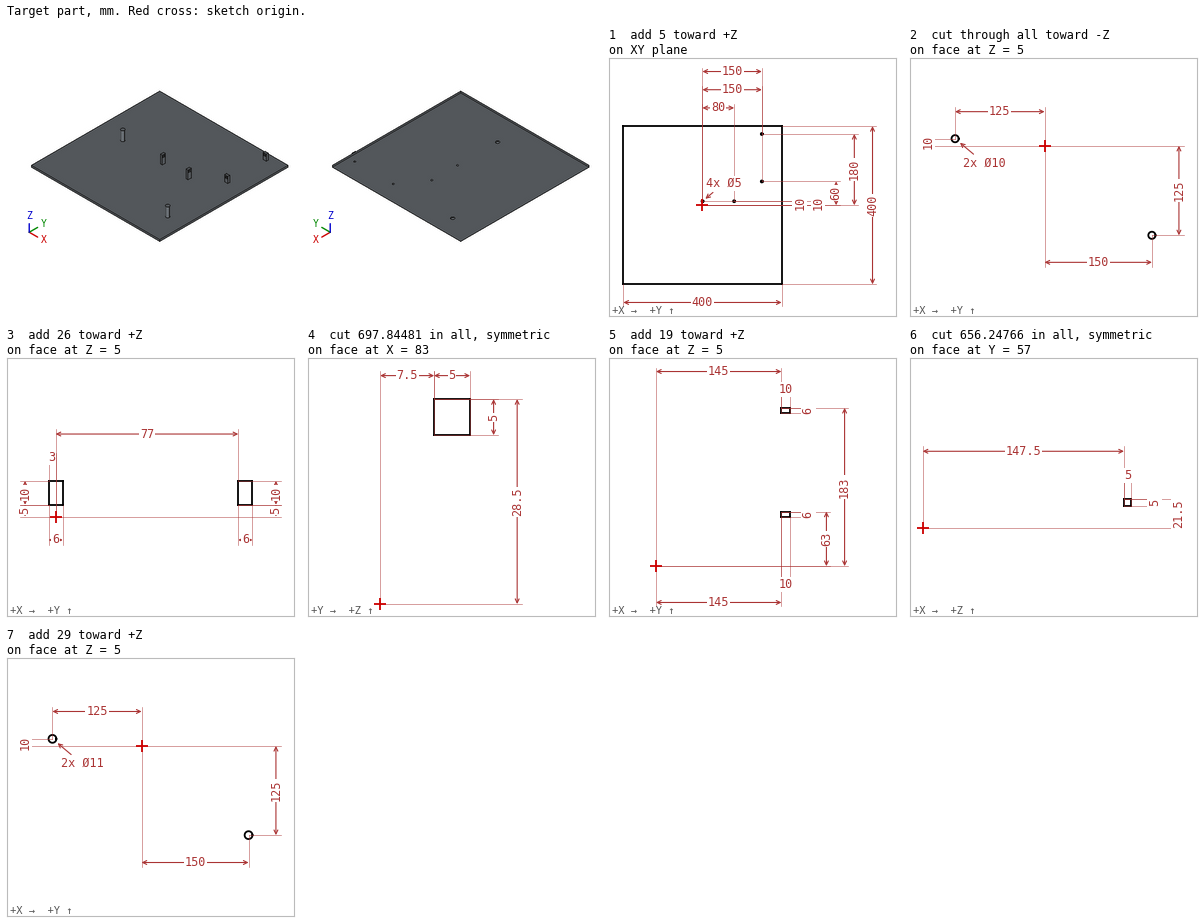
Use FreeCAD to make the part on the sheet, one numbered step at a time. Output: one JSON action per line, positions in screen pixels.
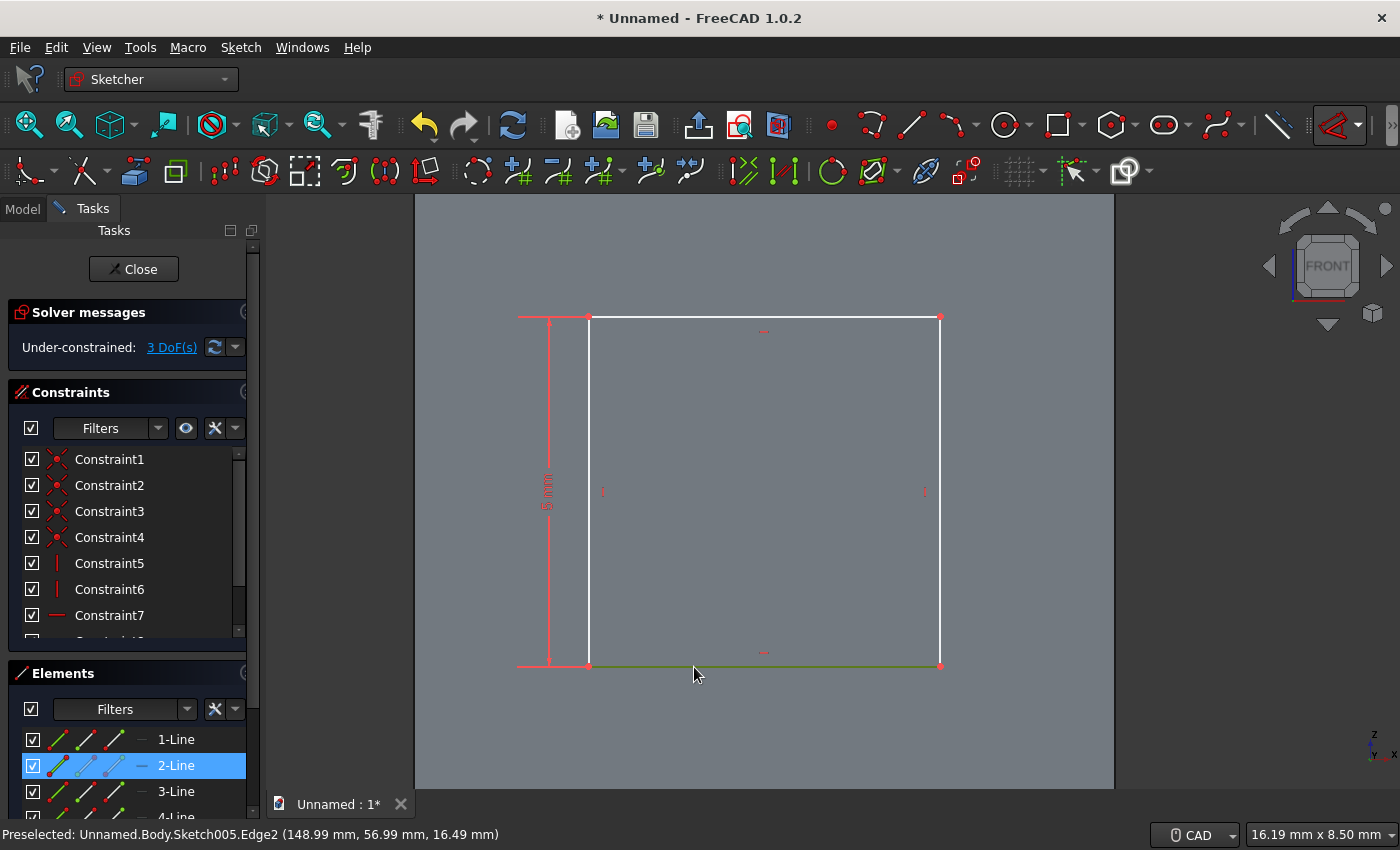
{"action": "left_click", "coordinate": [1360, 126]}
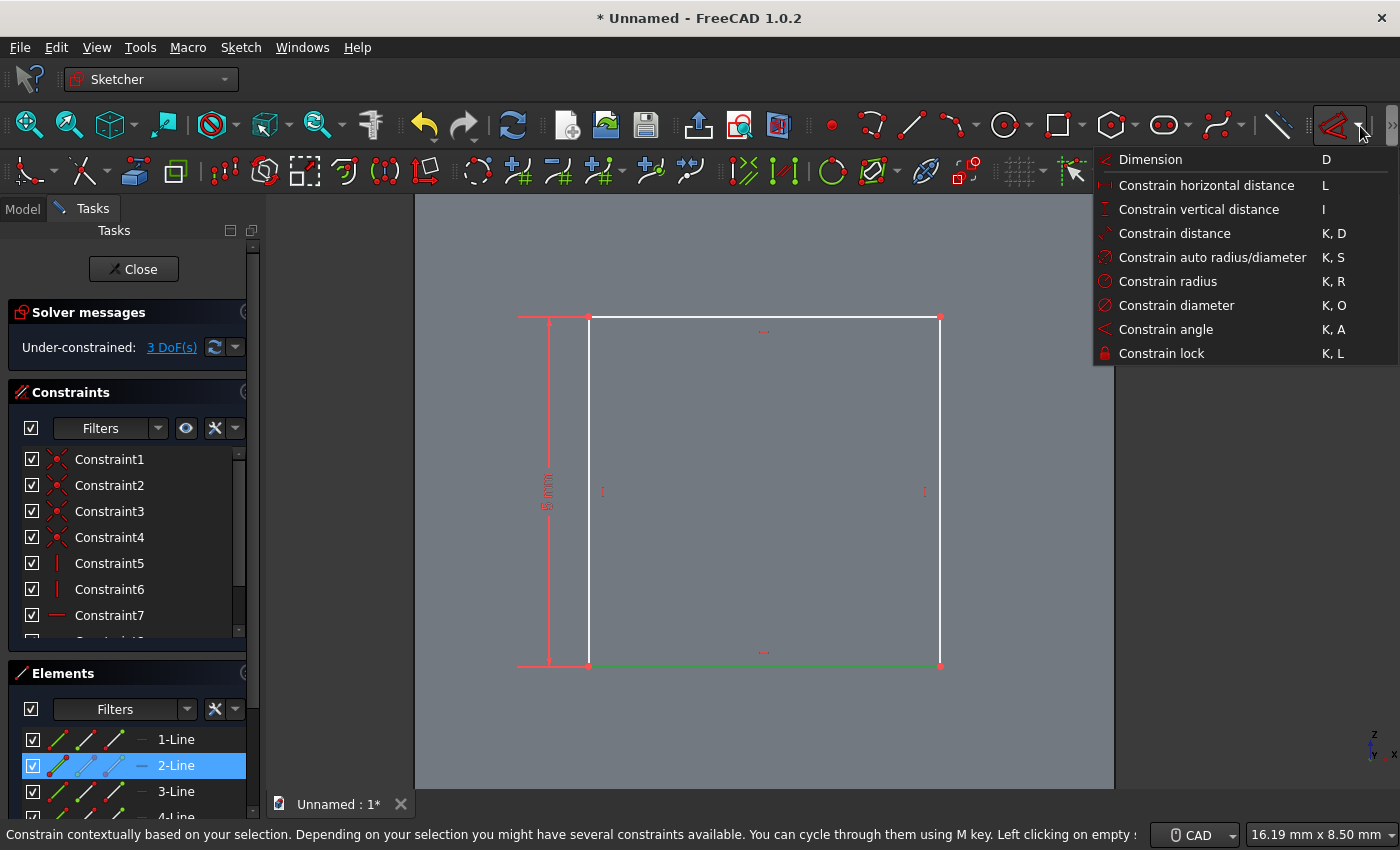
{"action": "left_click", "coordinate": [1246, 185]}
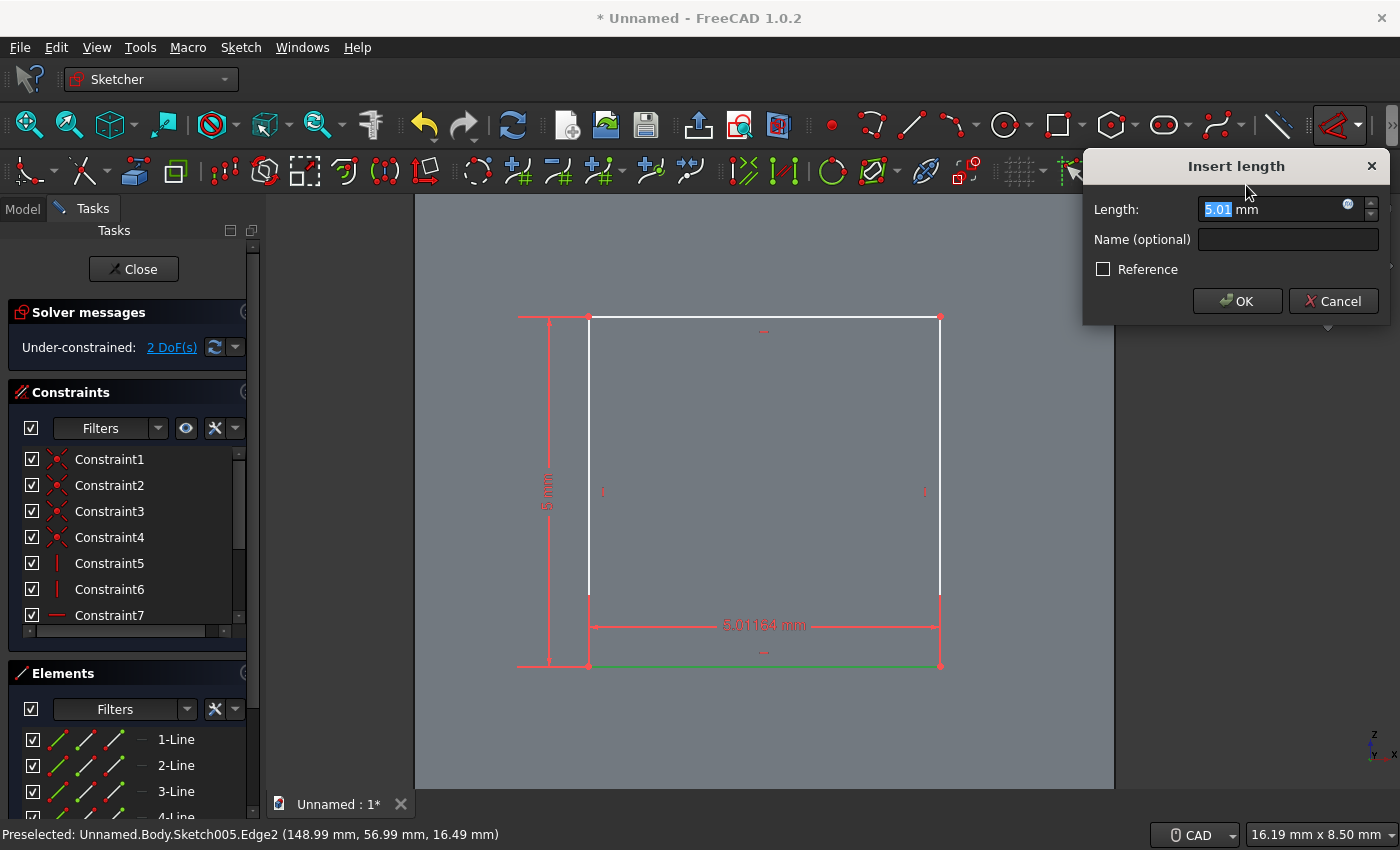
{"action": "type", "text": "5"}
{"action": "key", "text": "Return"}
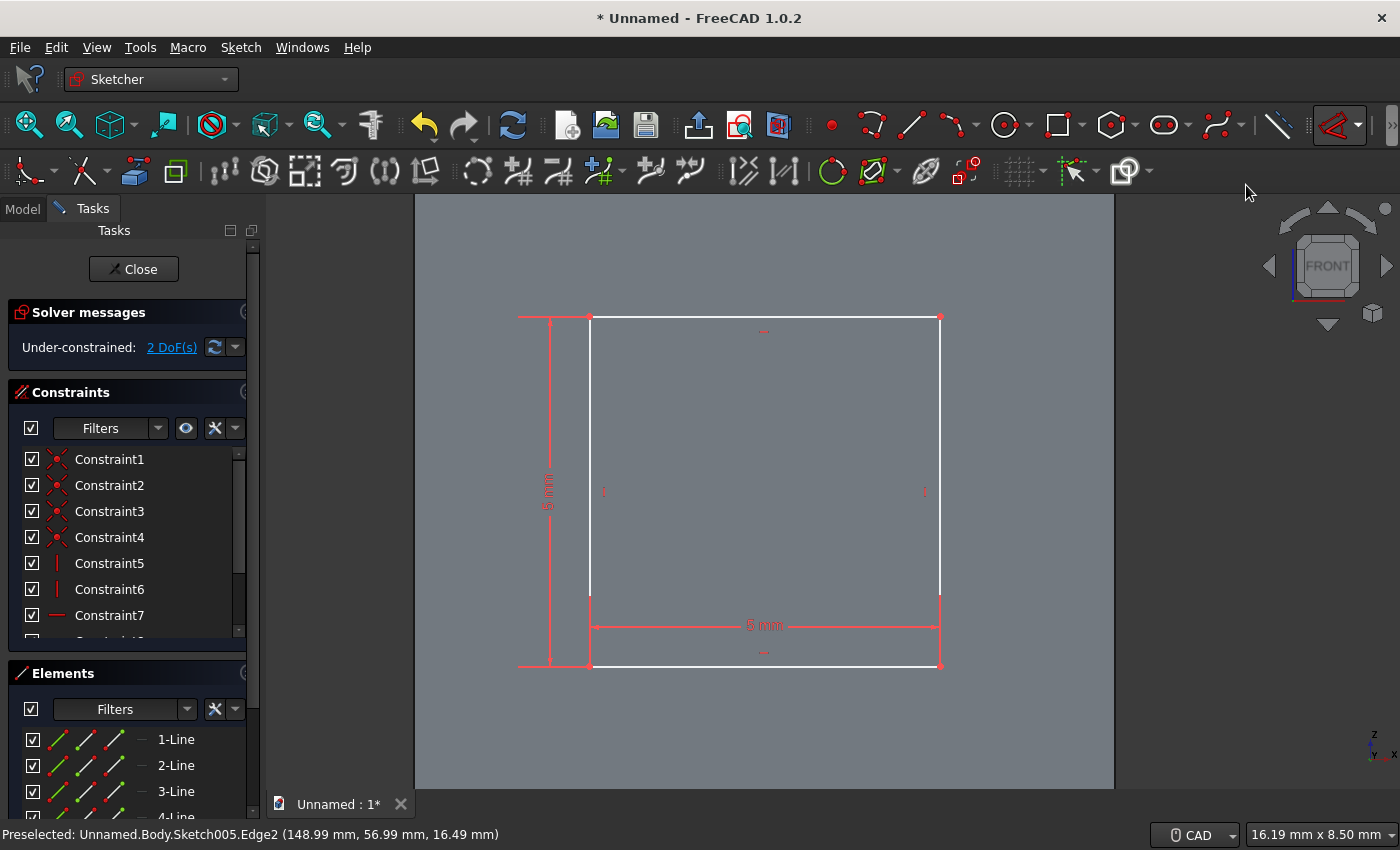
{"action": "left_click", "coordinate": [590, 317]}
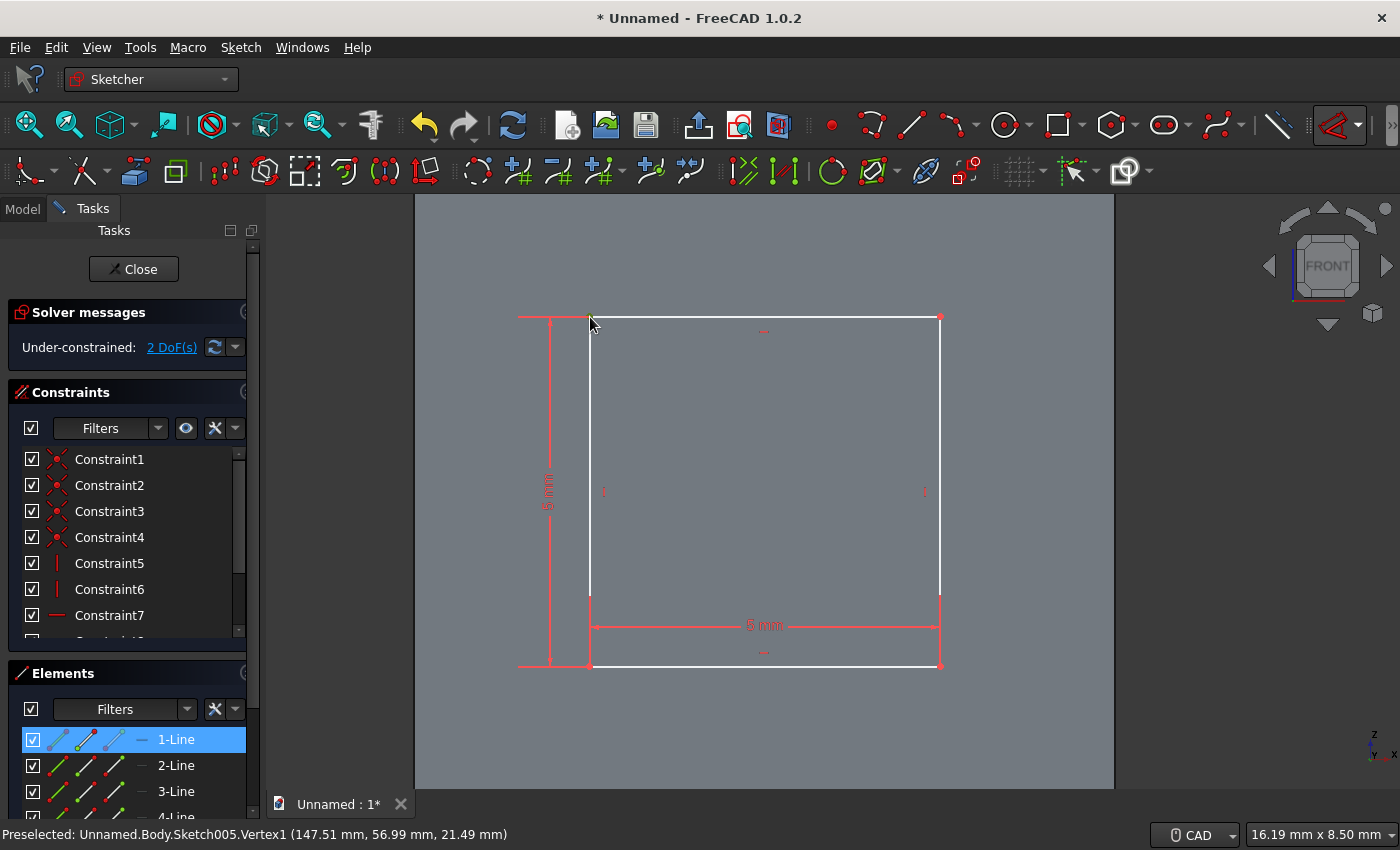
{"action": "key", "text": "i"}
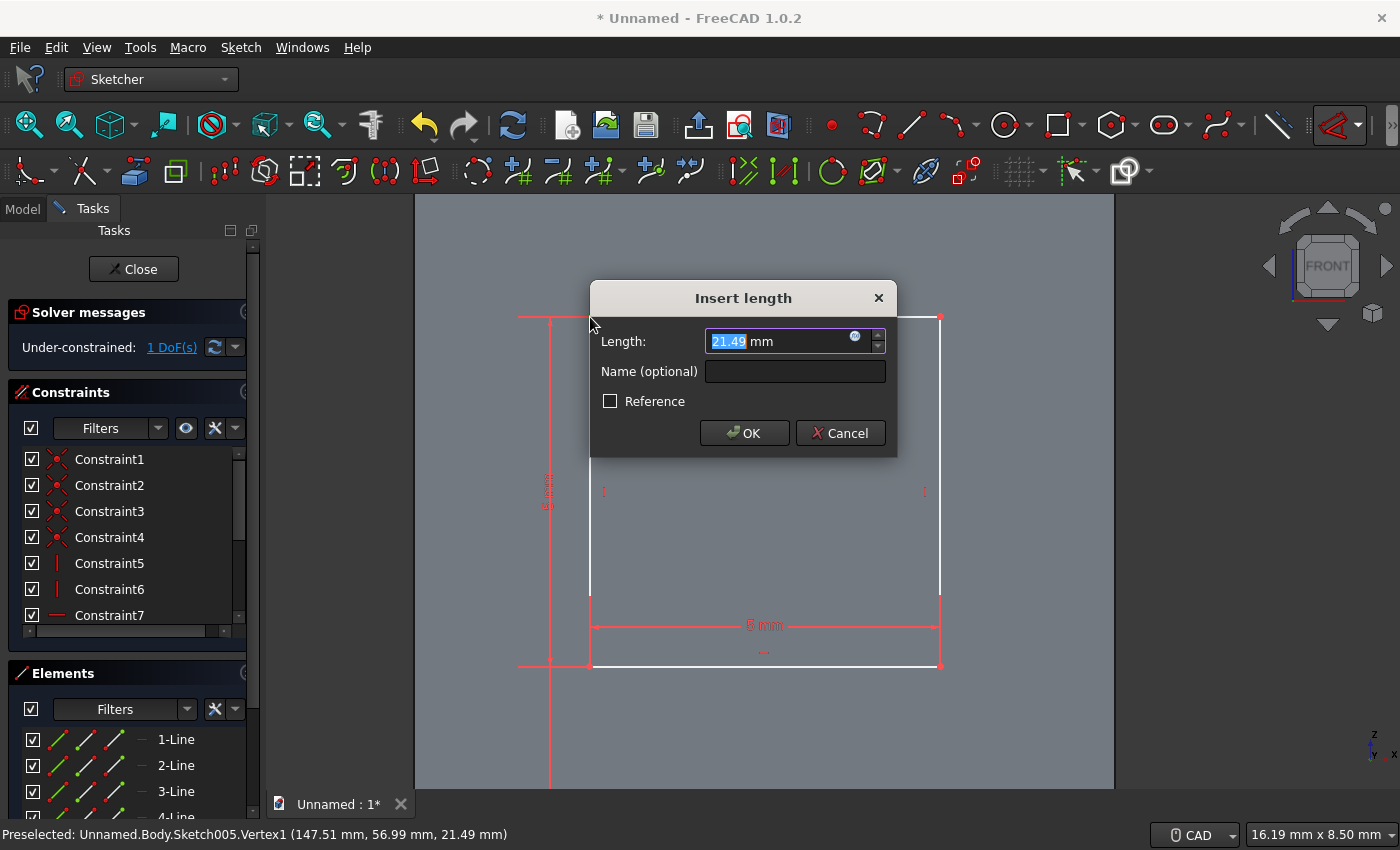
{"action": "type", "text": "21.5"}
{"action": "key", "text": "Return"}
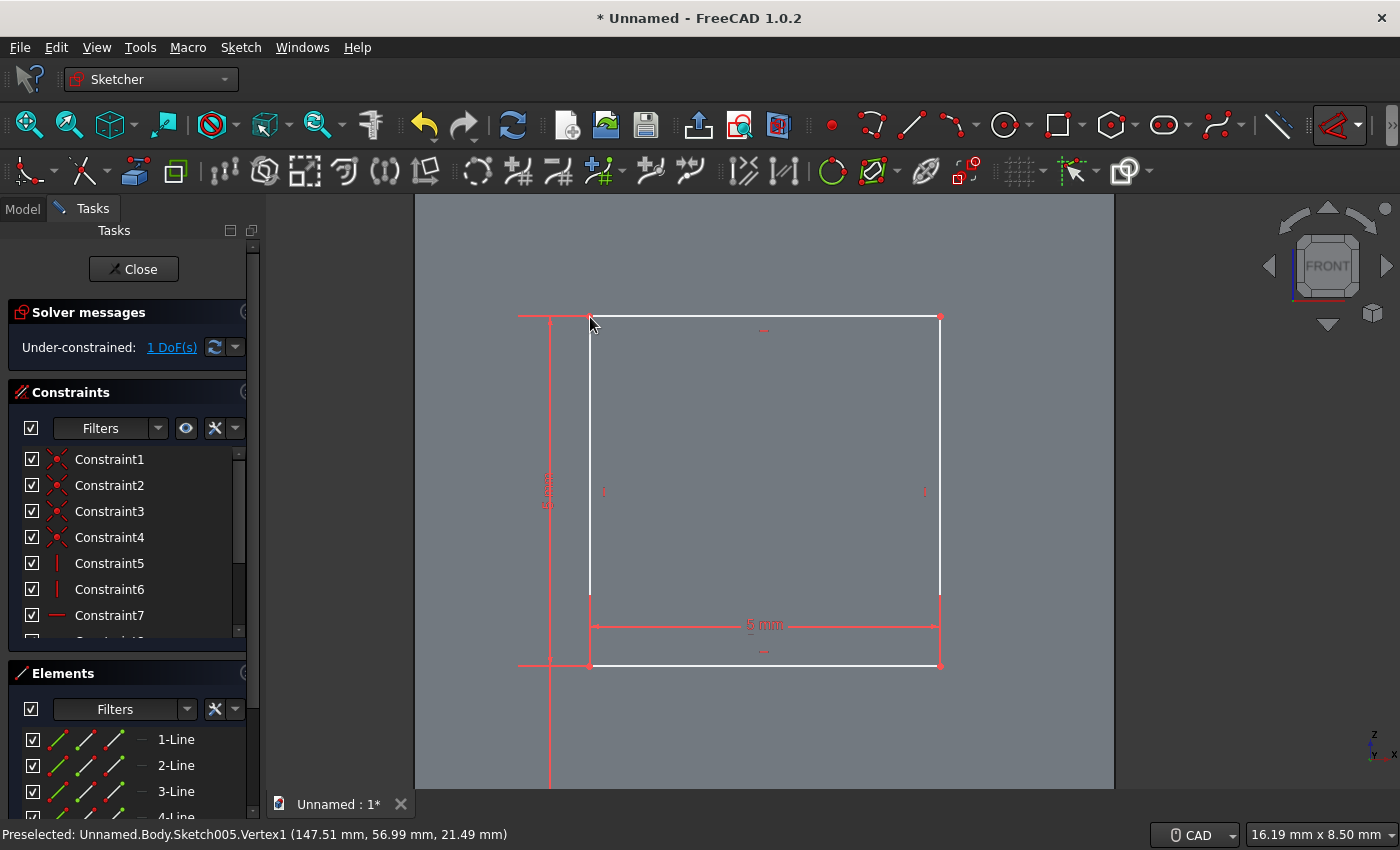
{"action": "left_click", "coordinate": [590, 316]}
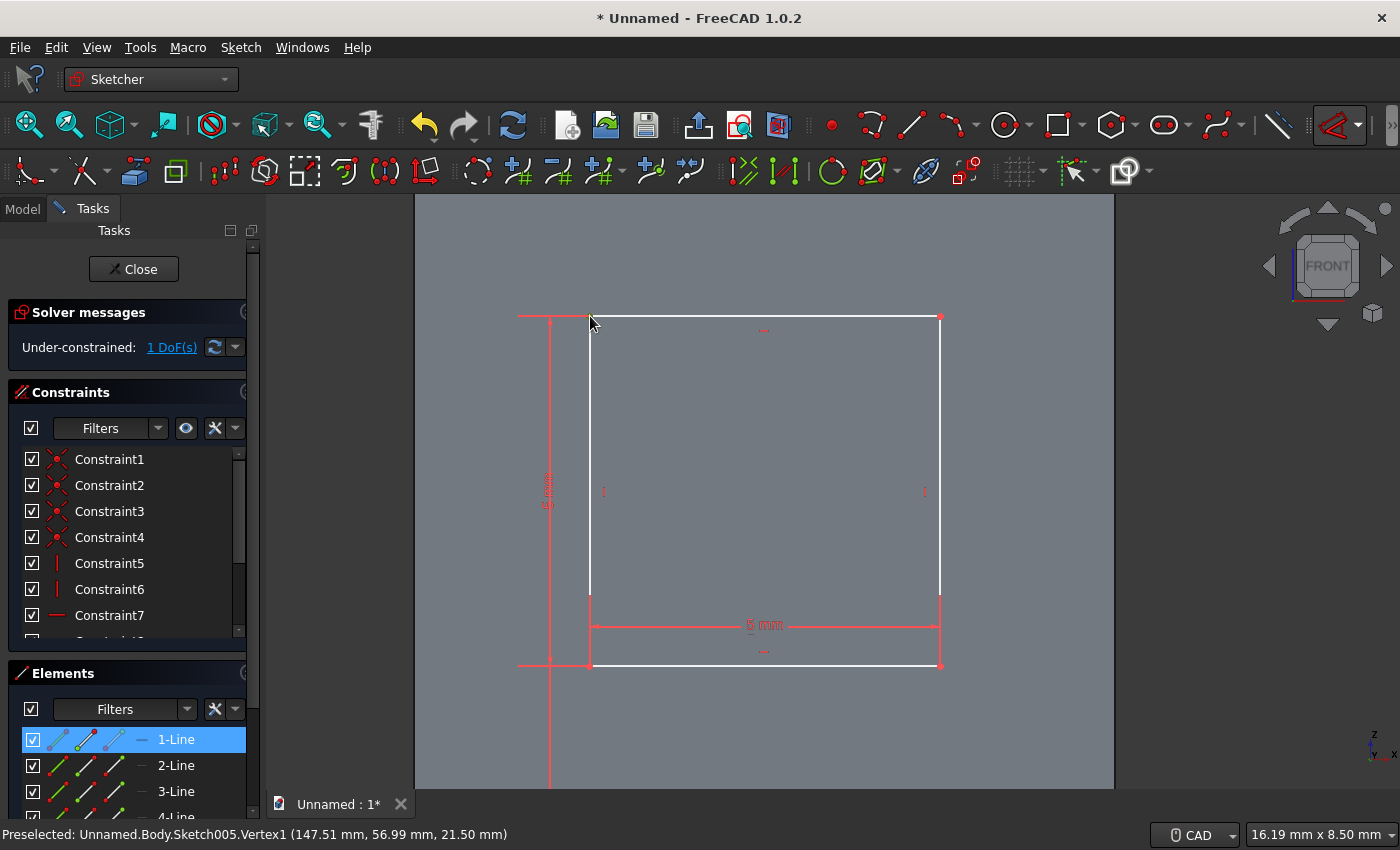
{"action": "key", "text": "l"}